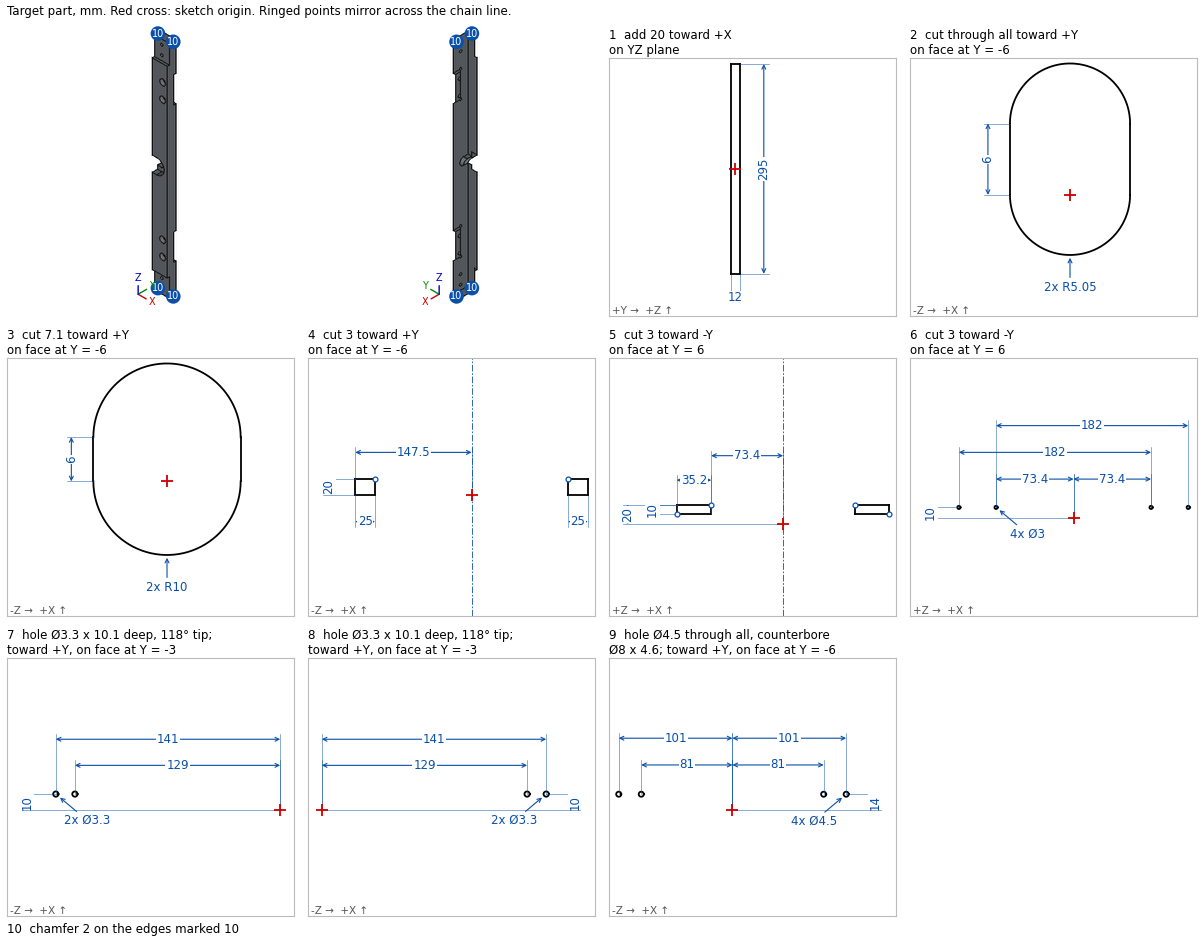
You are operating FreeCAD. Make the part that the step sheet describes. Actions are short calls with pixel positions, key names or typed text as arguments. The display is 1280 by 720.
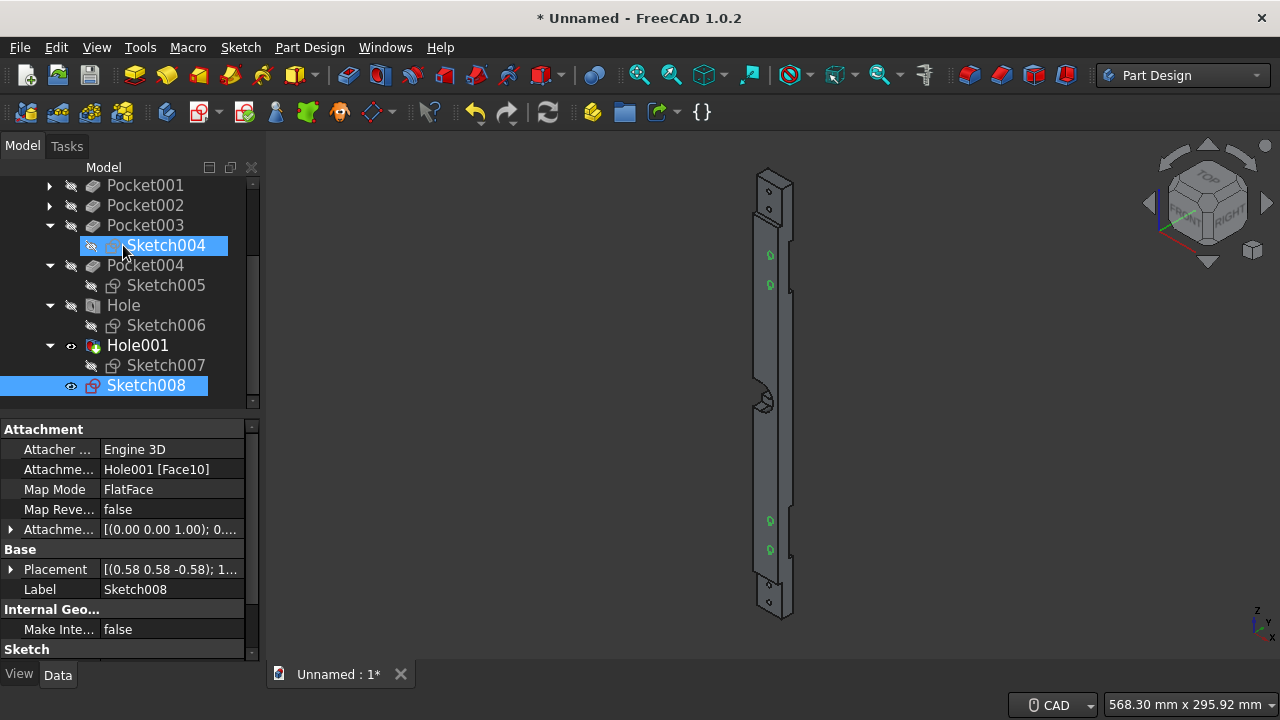
click(382, 76)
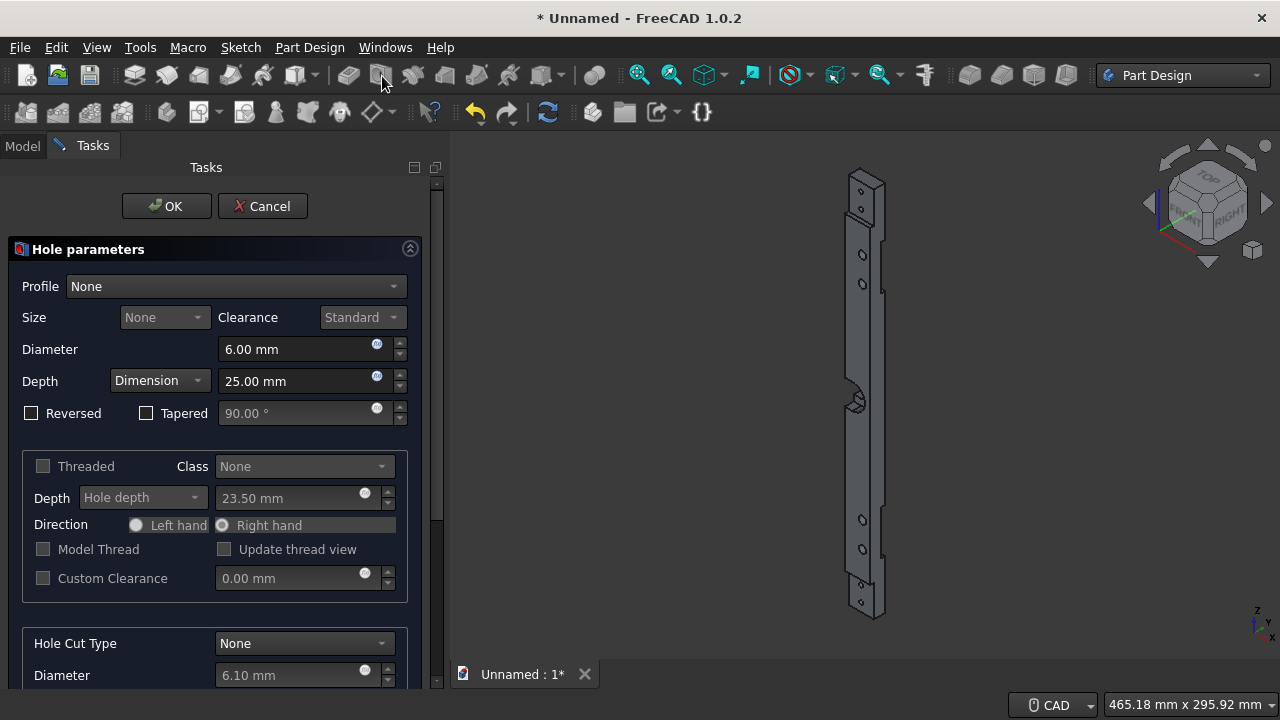
triple_click(305, 349)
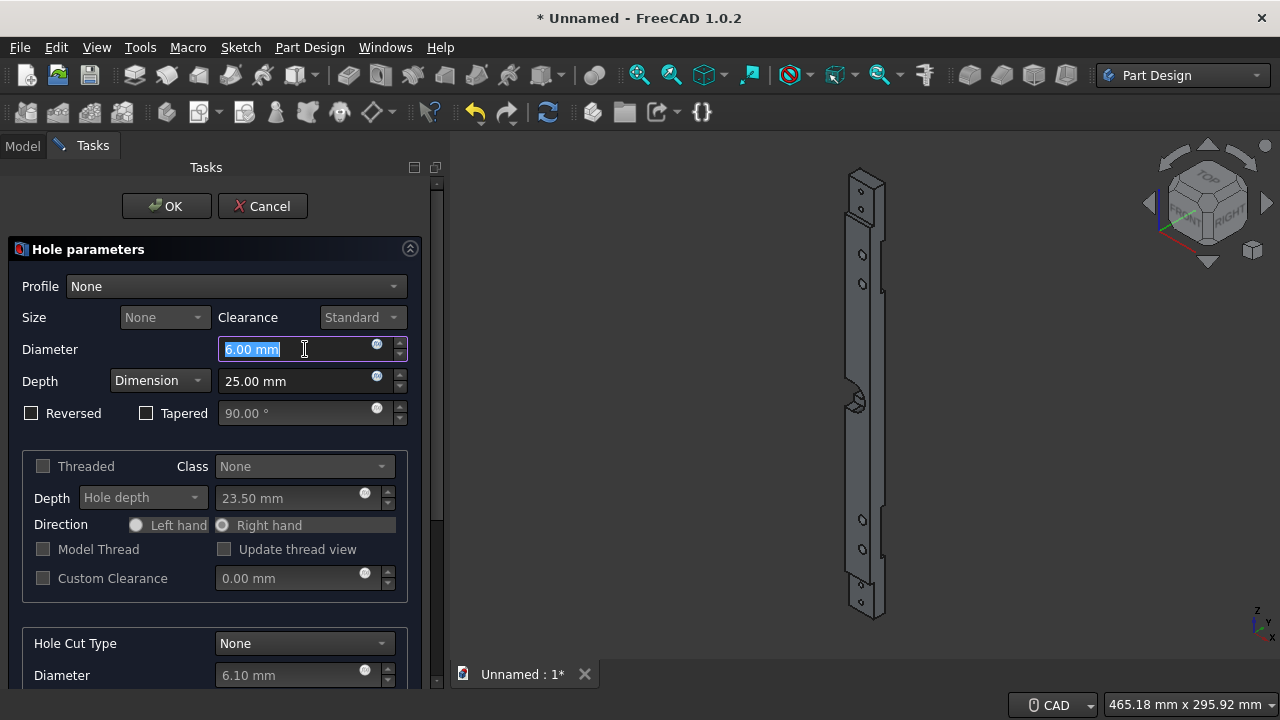
text(4.5)
key(Tab)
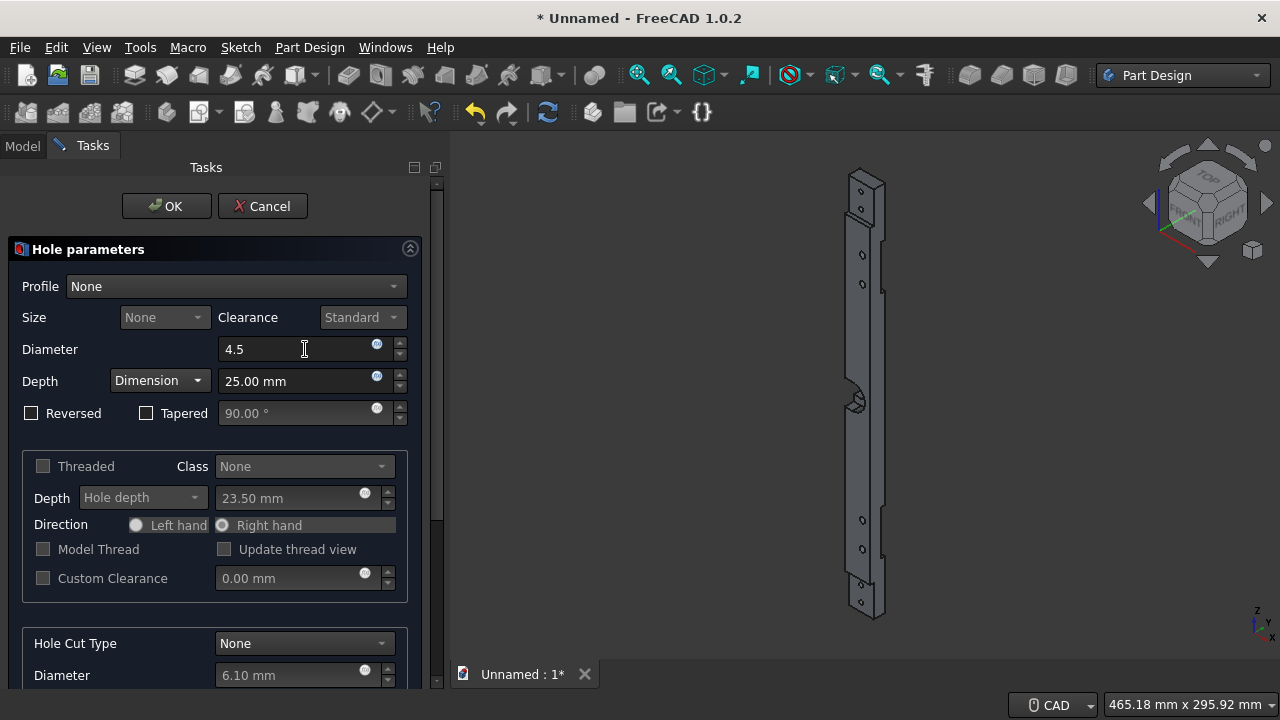
click(161, 380)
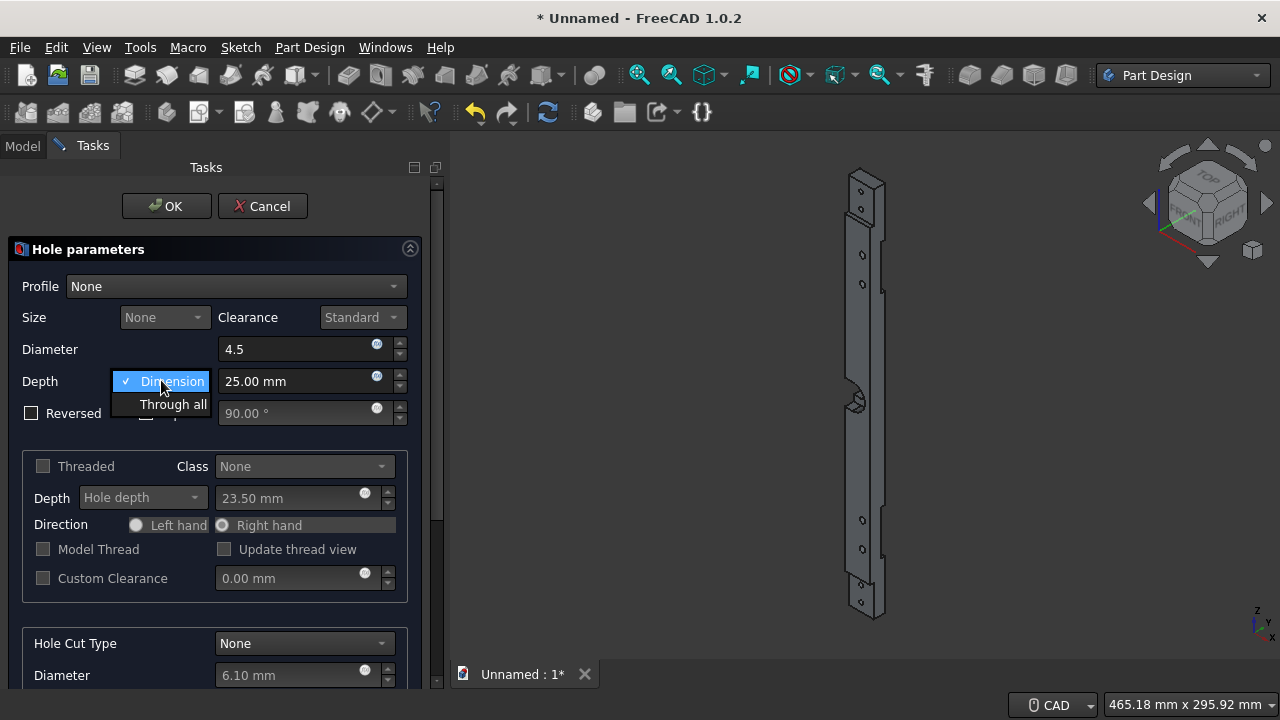
click(160, 404)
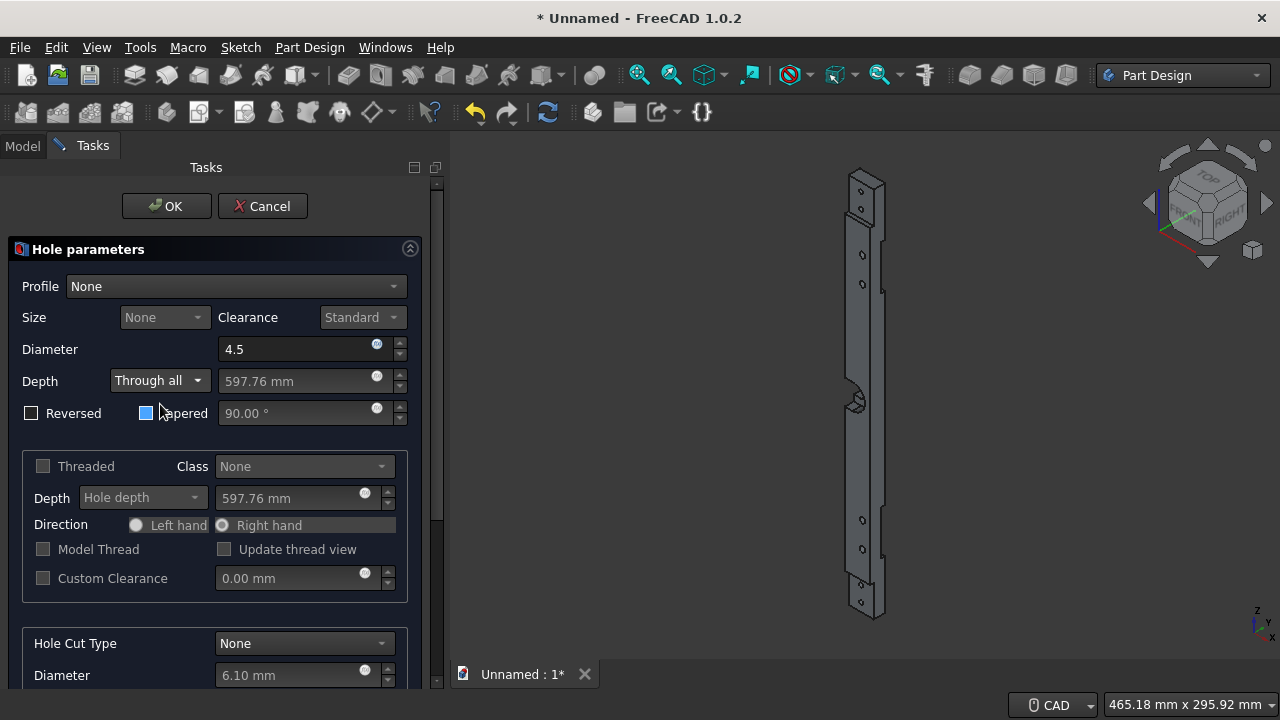
click(306, 644)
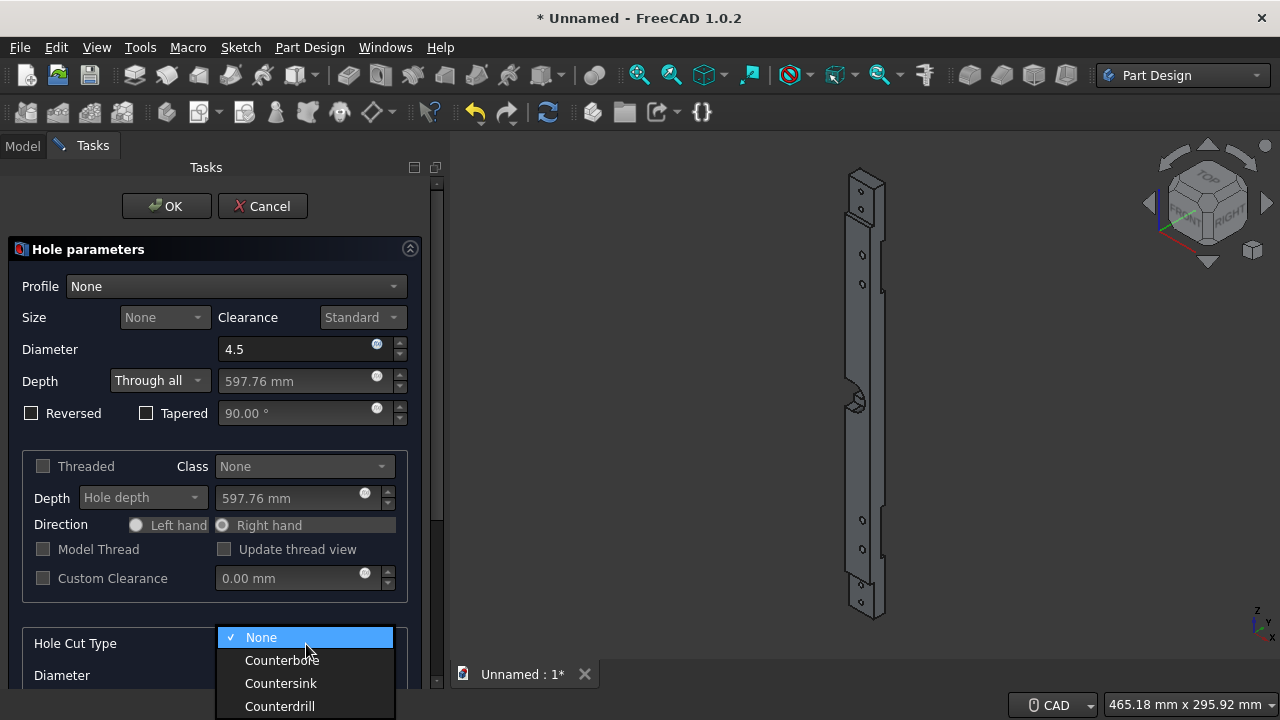
click(304, 660)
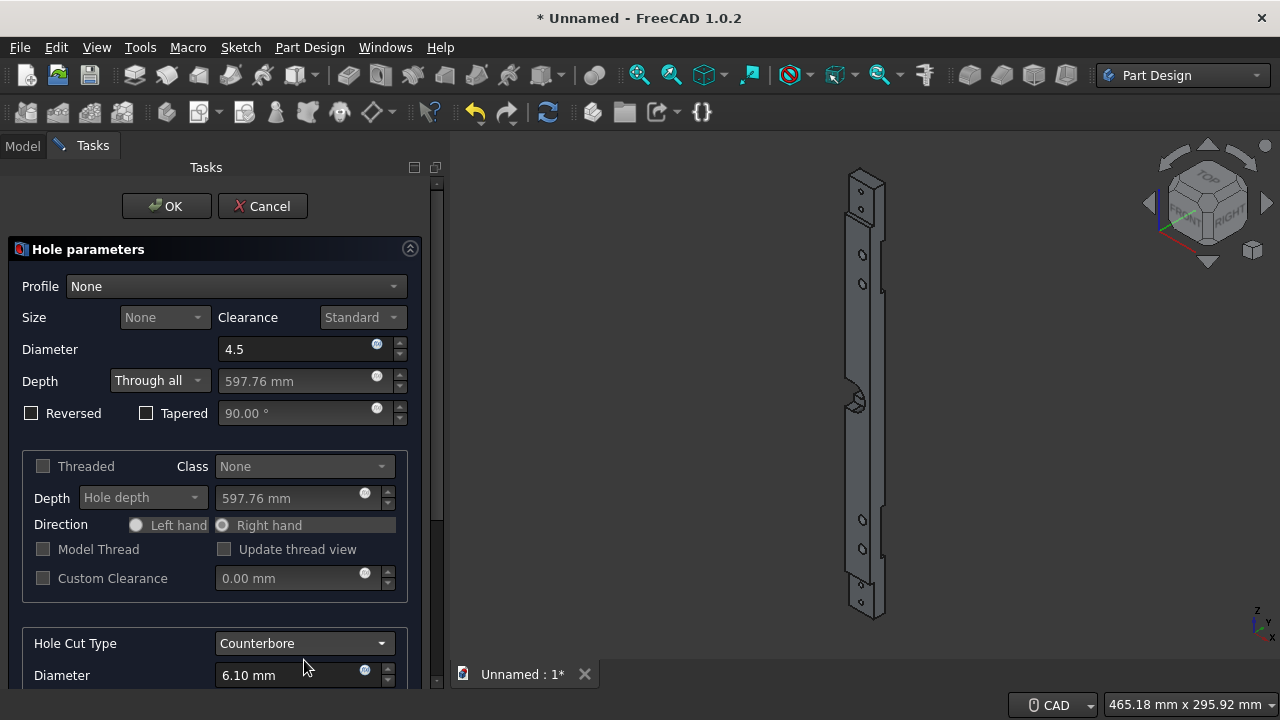
triple_click(298, 675)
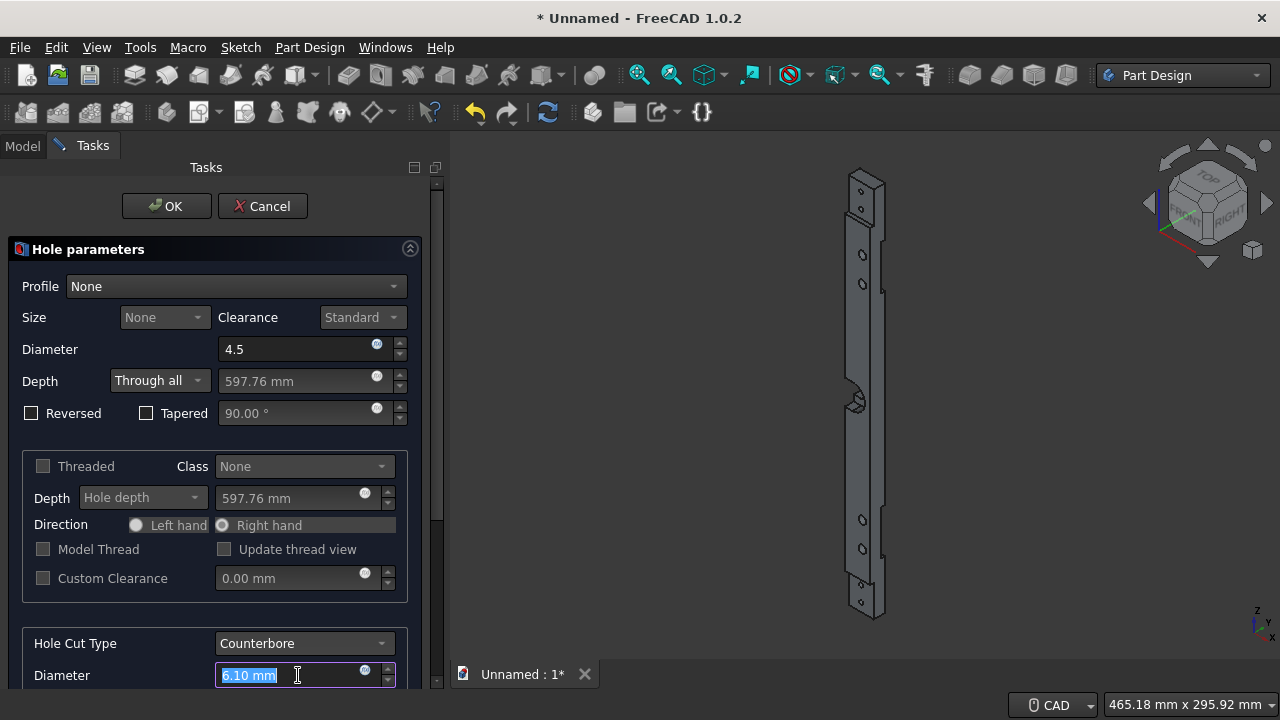
text(8)
key(Tab)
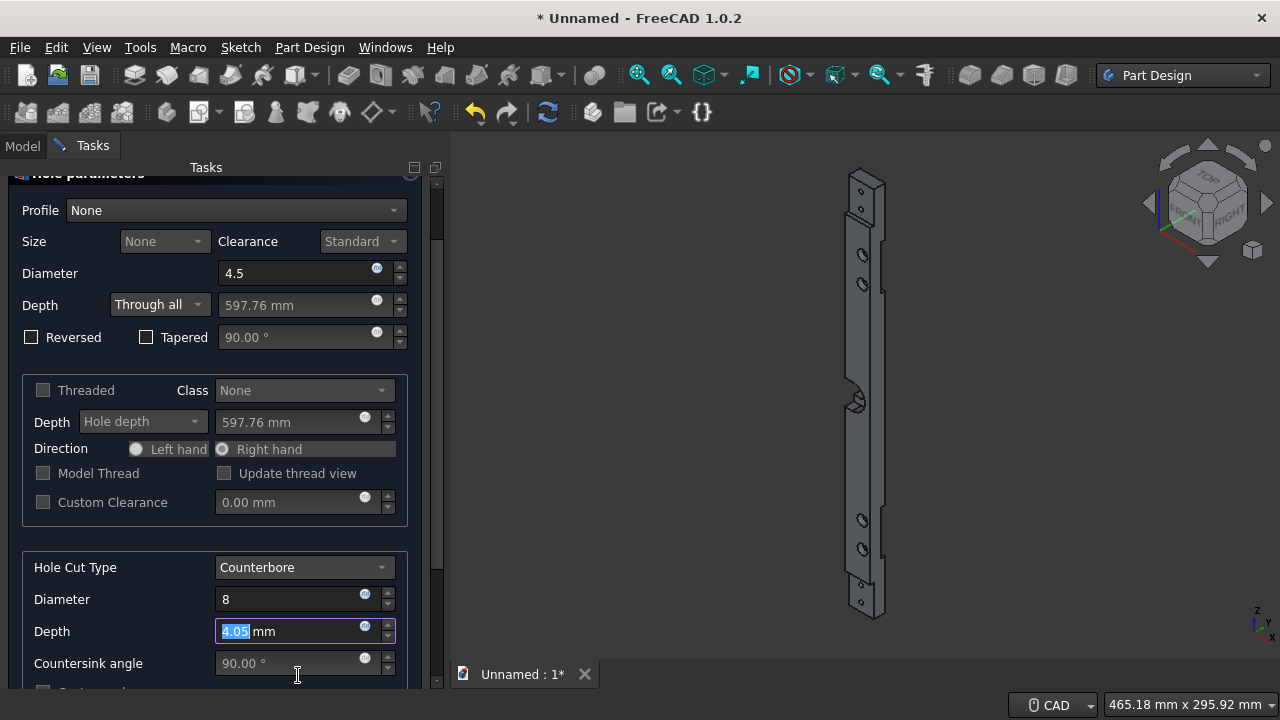
text(4.6)
key(Tab)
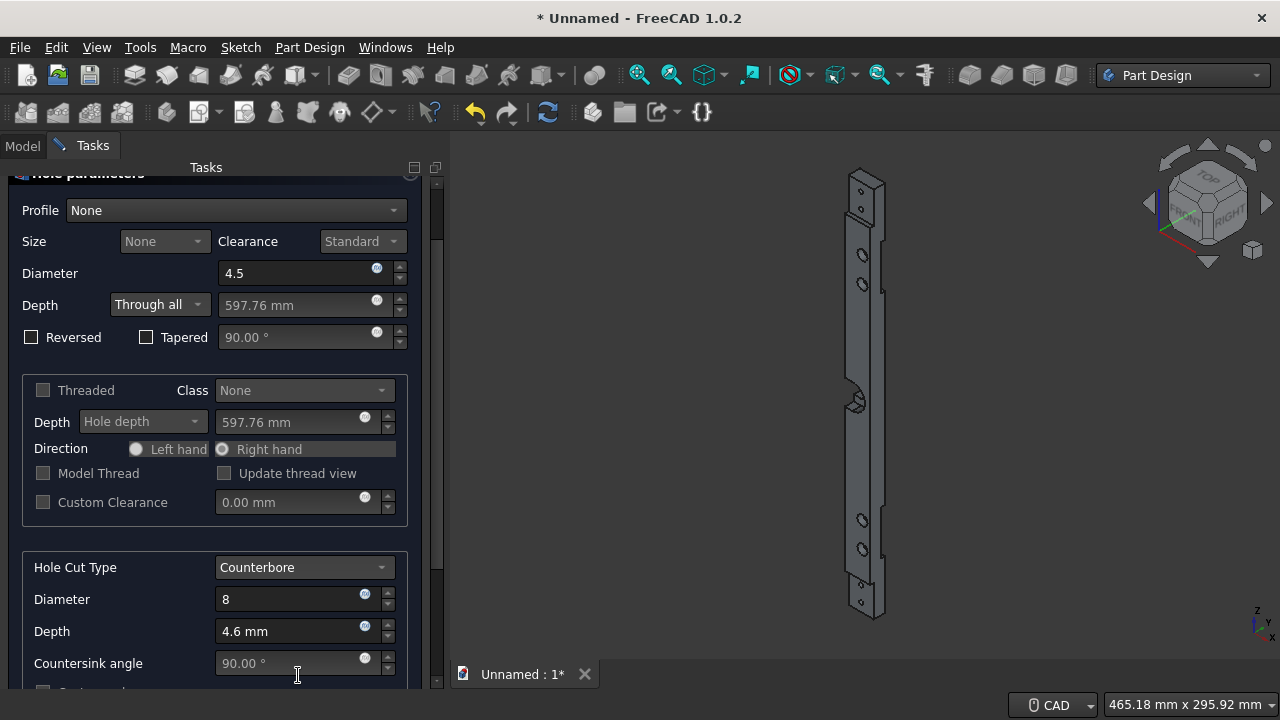
scroll(437, 432, up, 3)